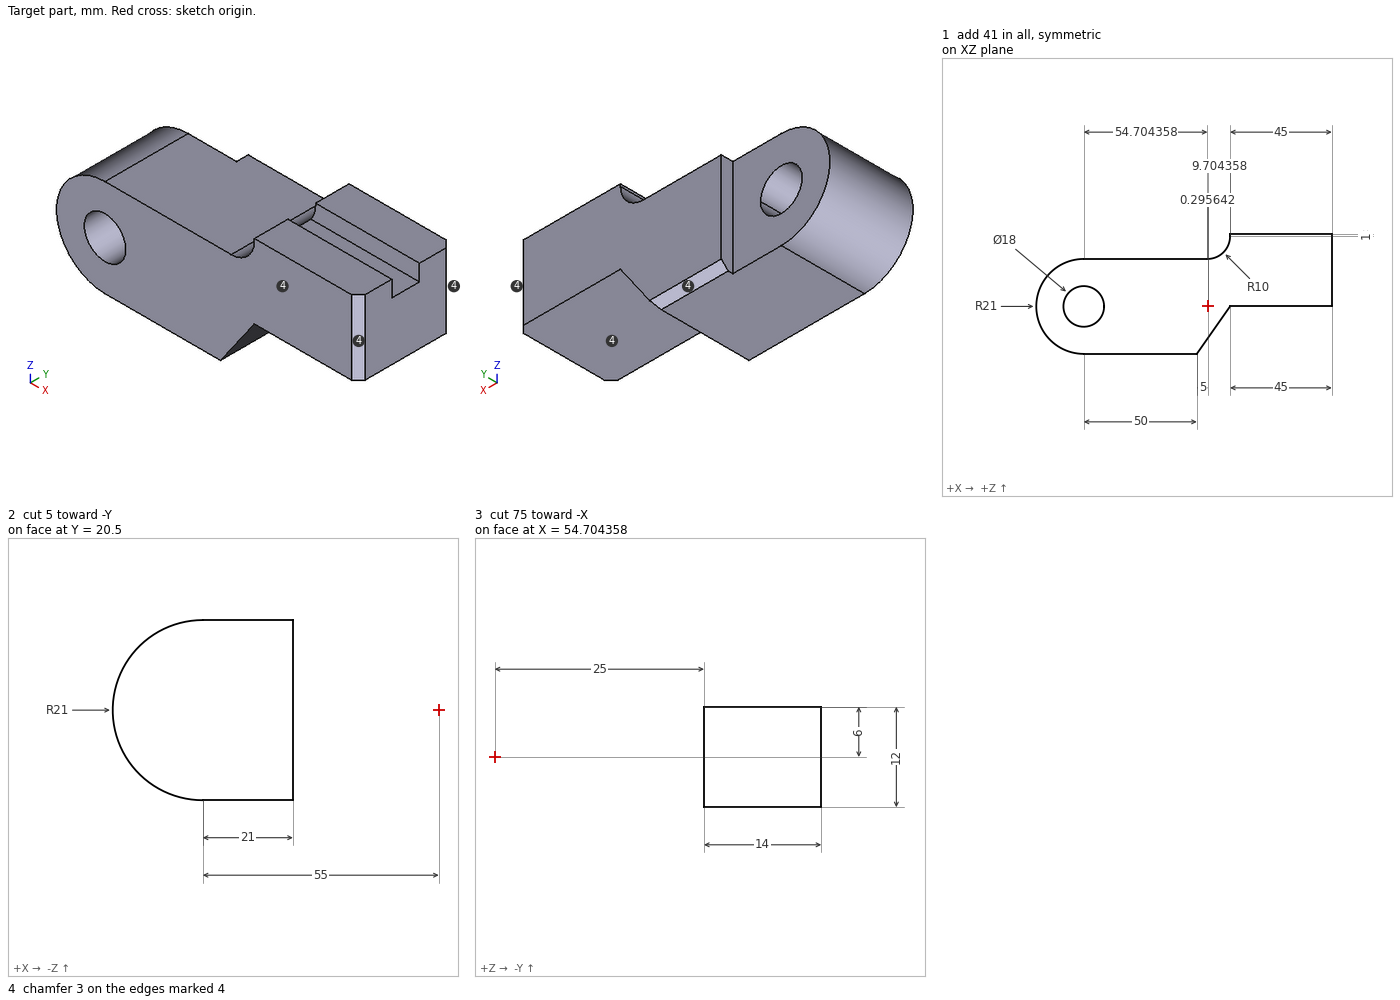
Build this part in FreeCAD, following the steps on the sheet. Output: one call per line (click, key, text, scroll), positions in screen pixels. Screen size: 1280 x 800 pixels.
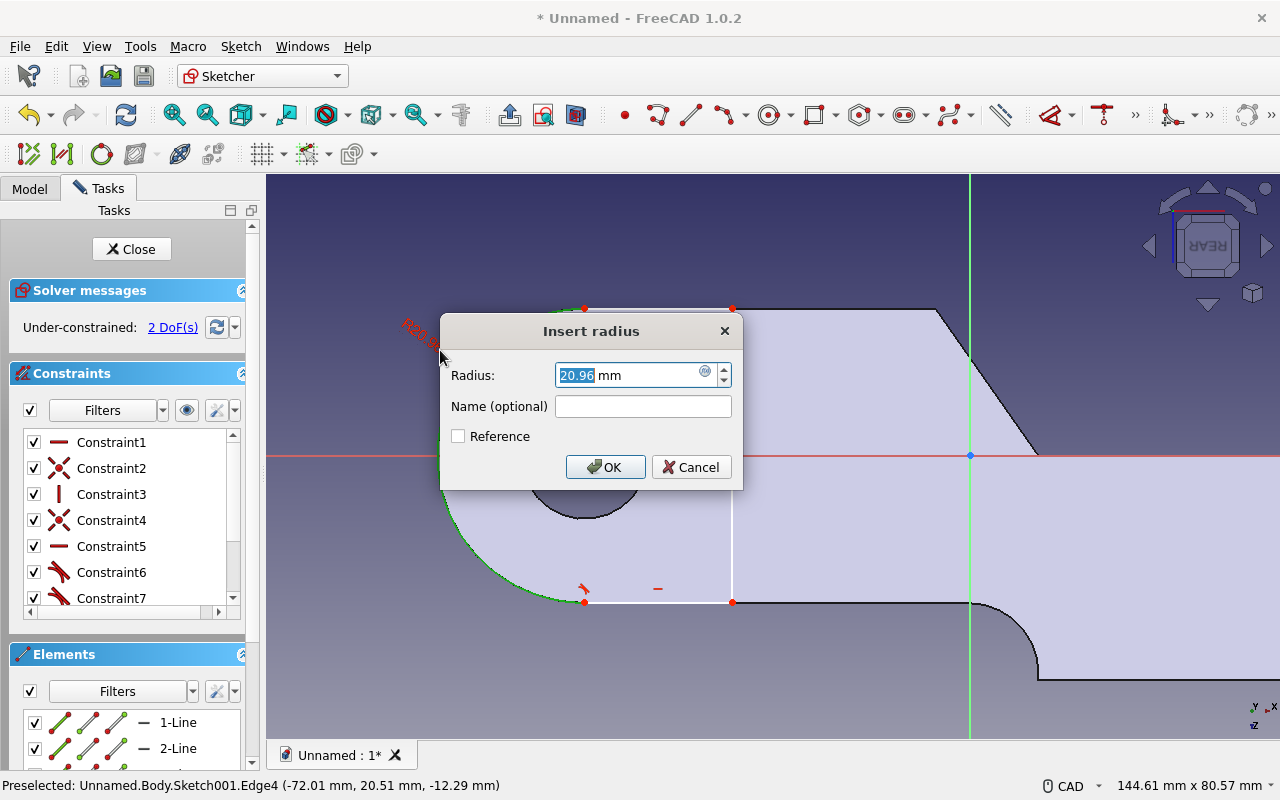
text(21)
key(Return)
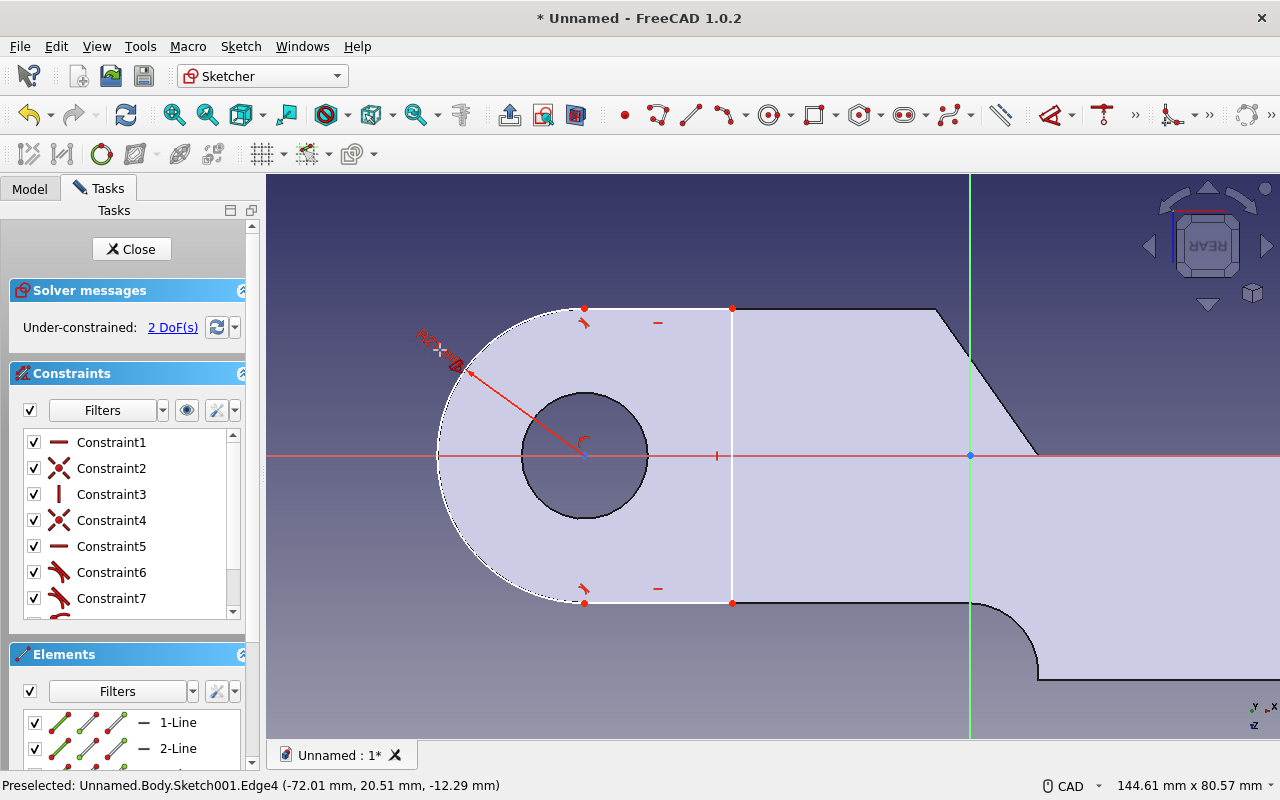
click(629, 603)
click(658, 637)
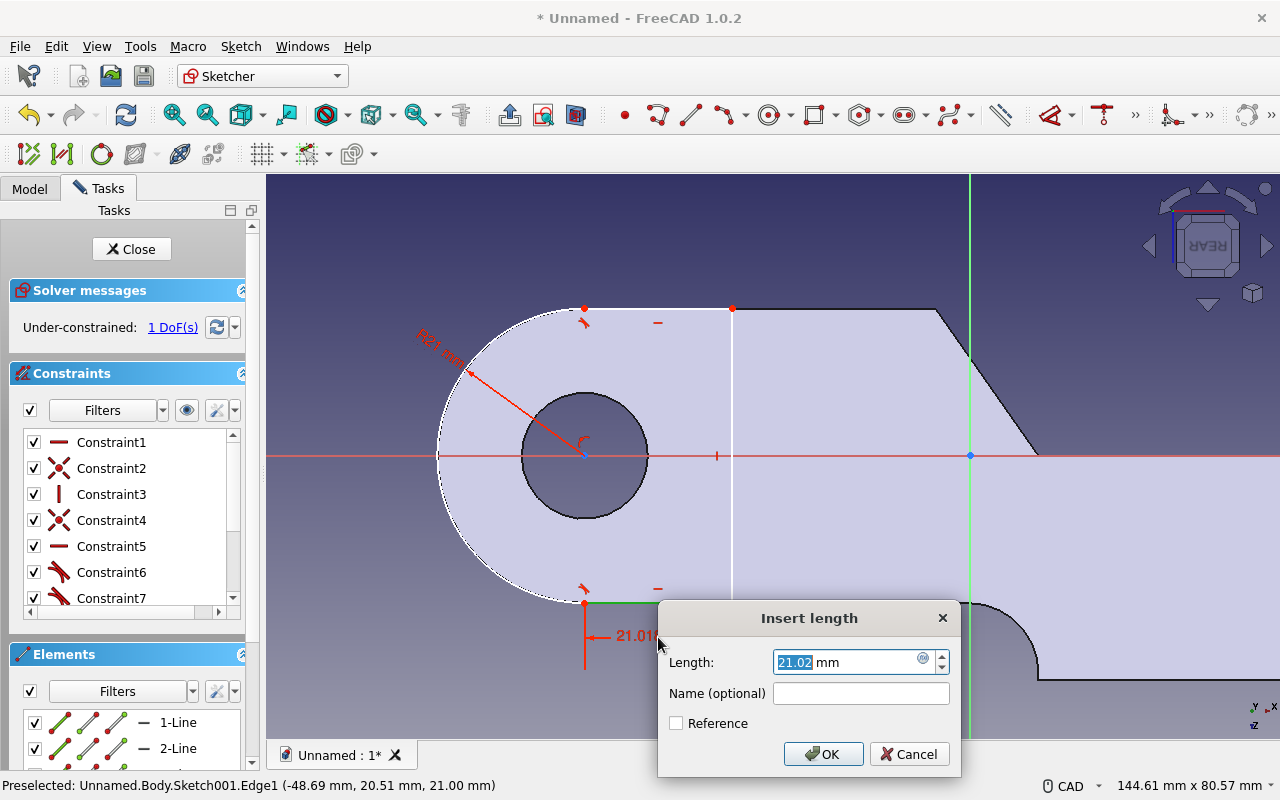
text(21)
key(Return)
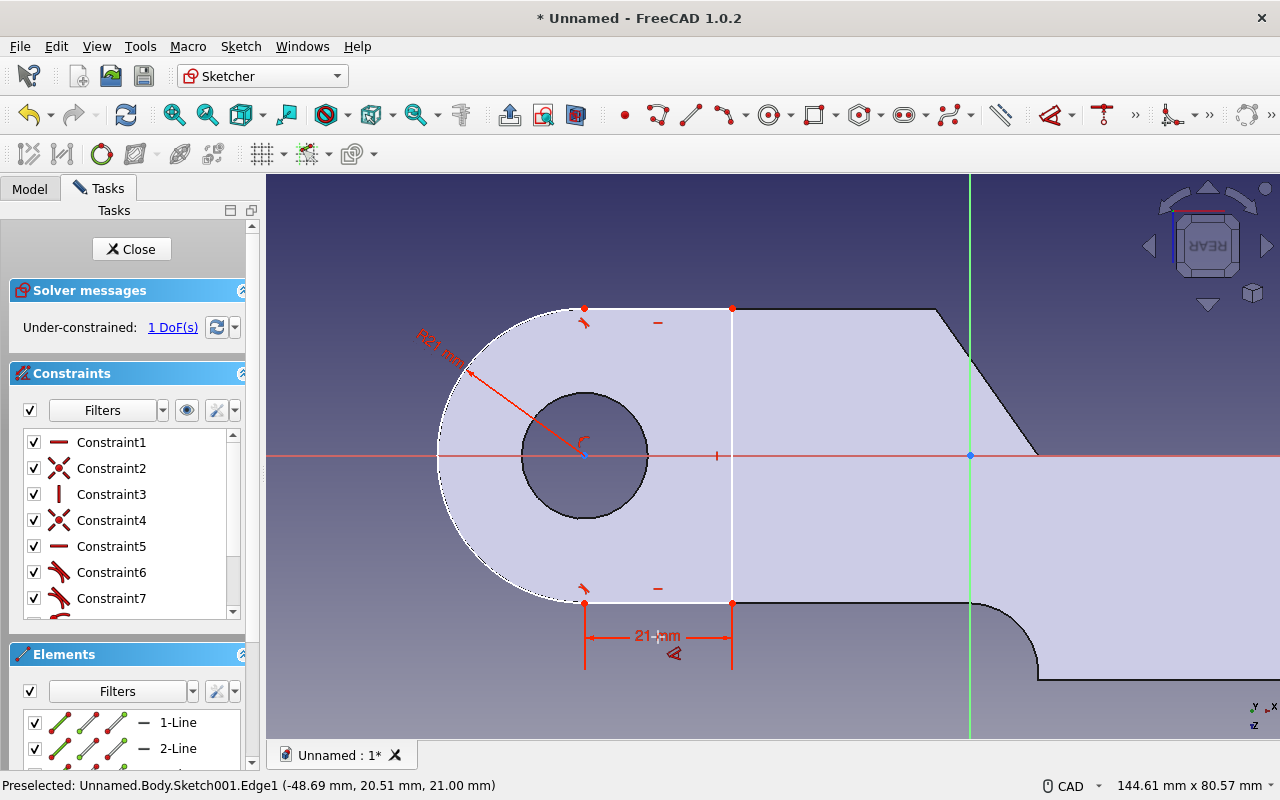
click(585, 603)
click(778, 637)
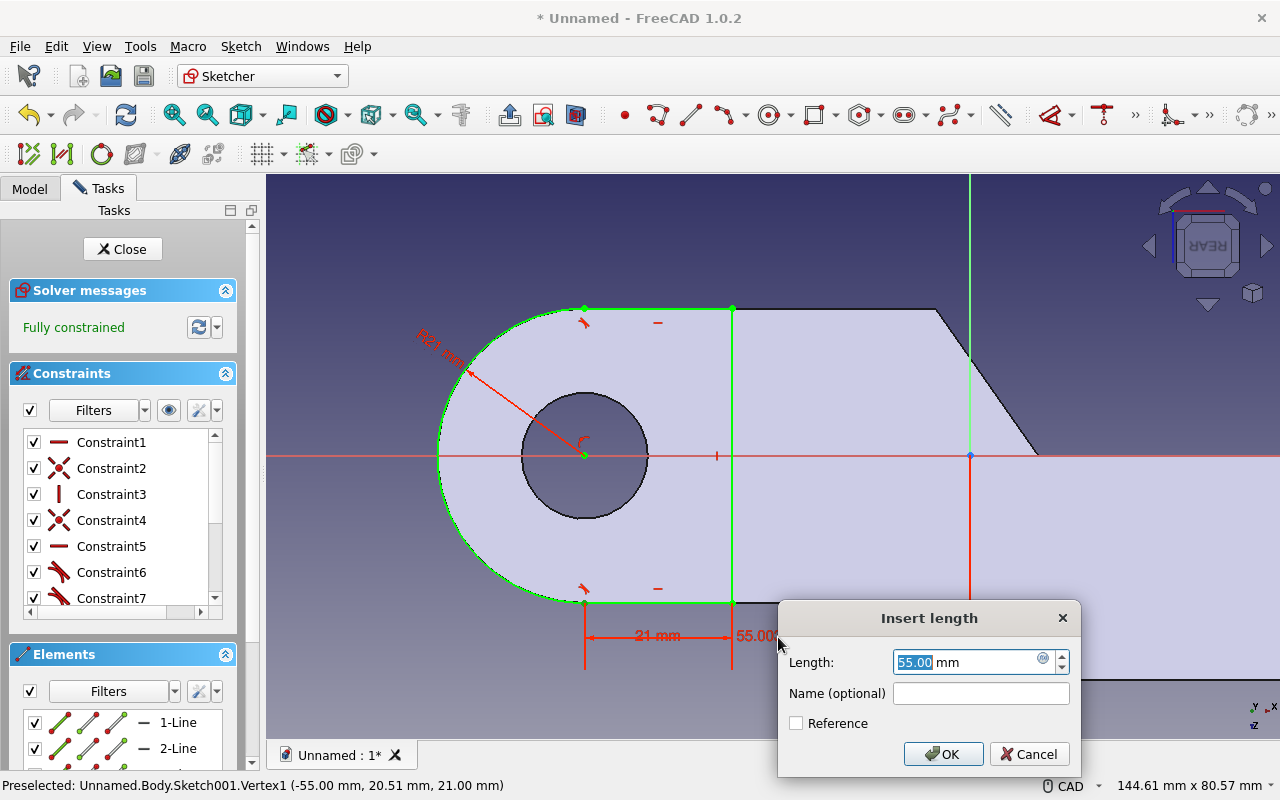
text(55)
key(Return)
key(Escape)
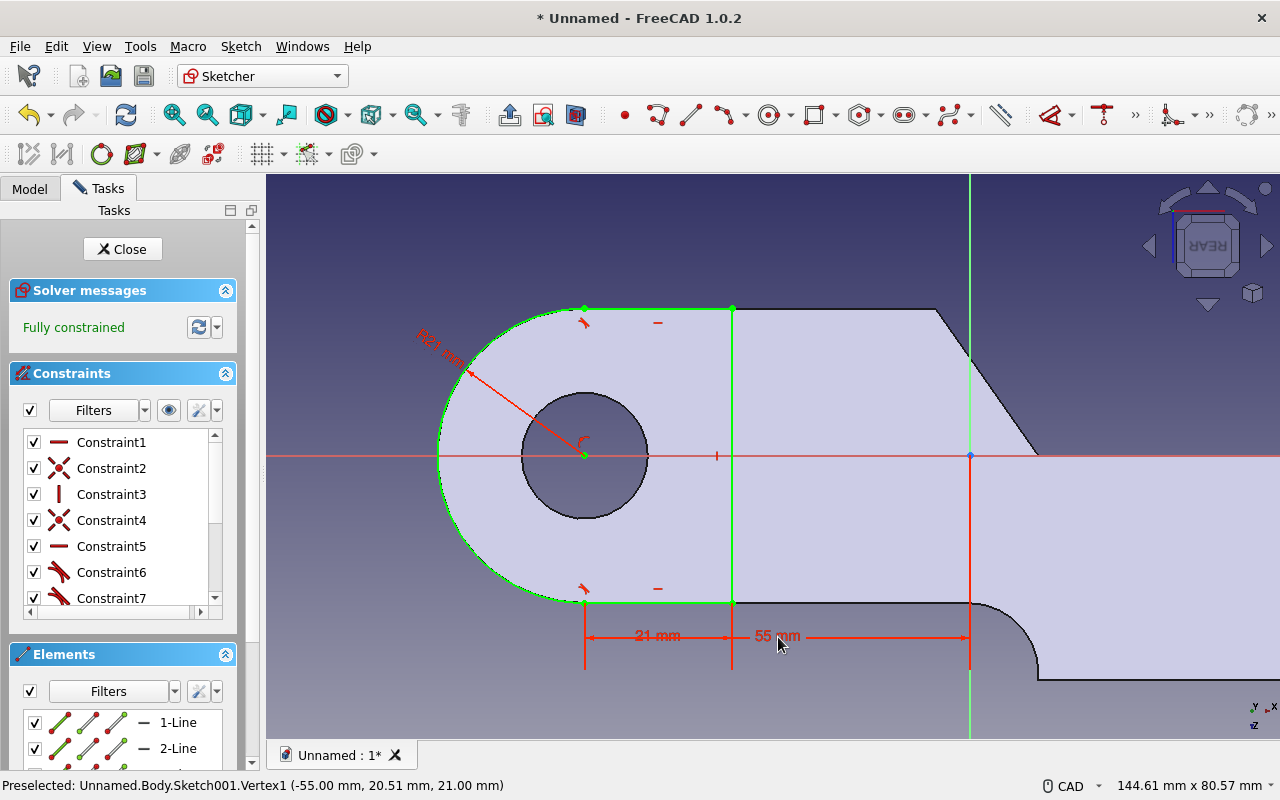
click(123, 249)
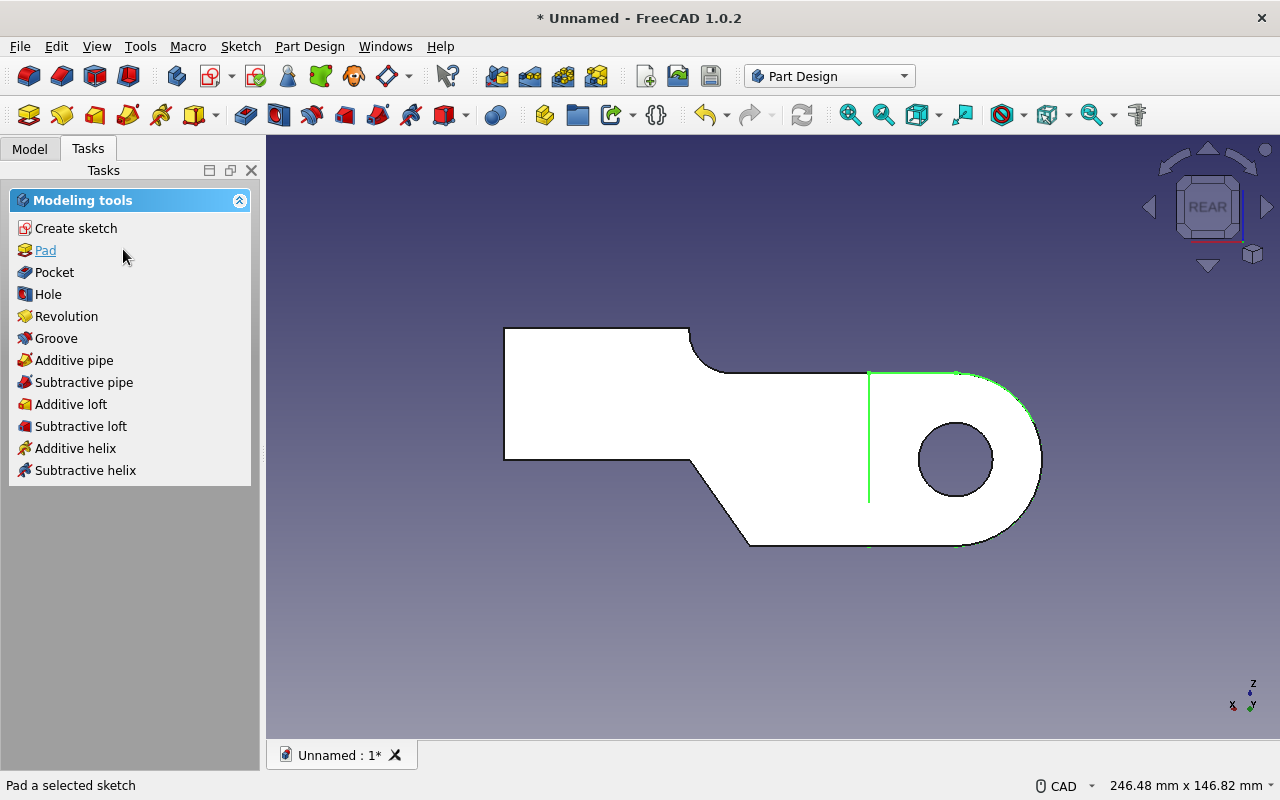
click(246, 116)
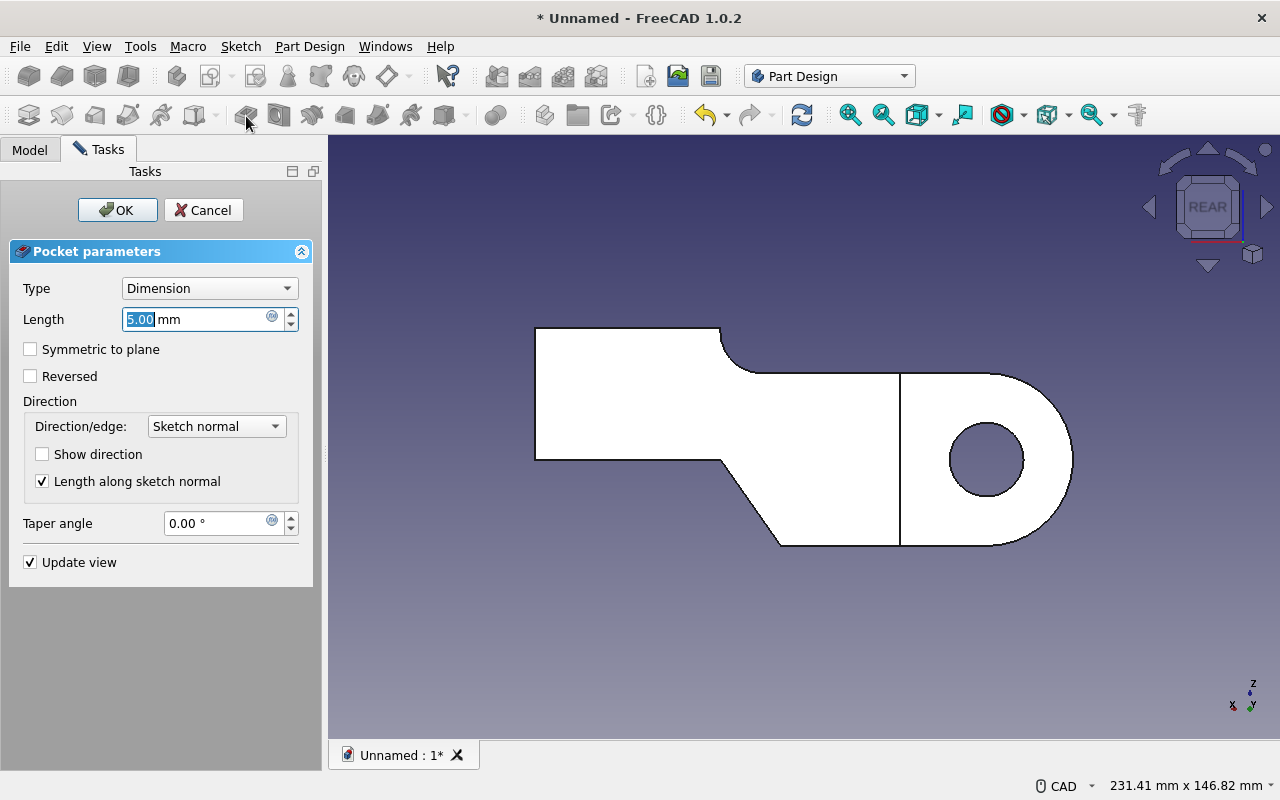
text(5)
key(Tab)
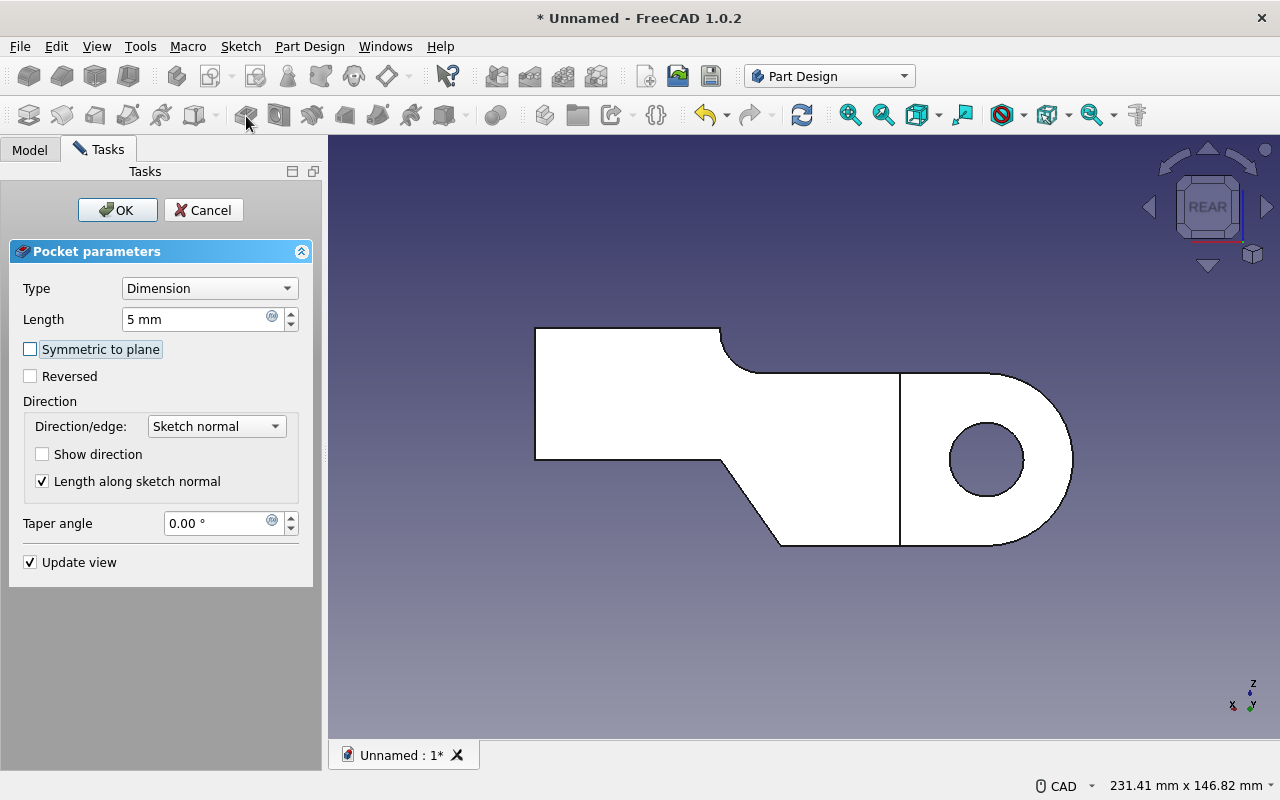
click(118, 210)